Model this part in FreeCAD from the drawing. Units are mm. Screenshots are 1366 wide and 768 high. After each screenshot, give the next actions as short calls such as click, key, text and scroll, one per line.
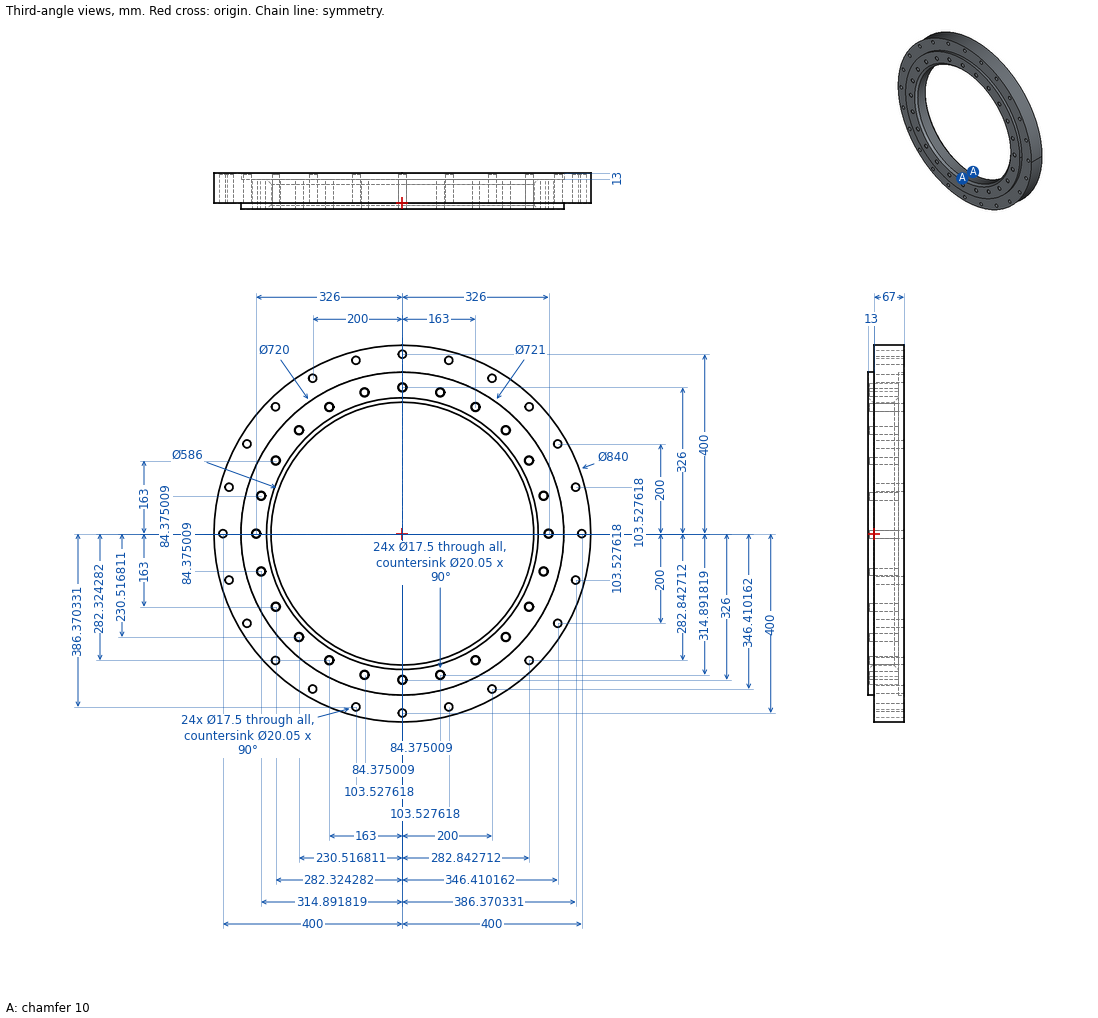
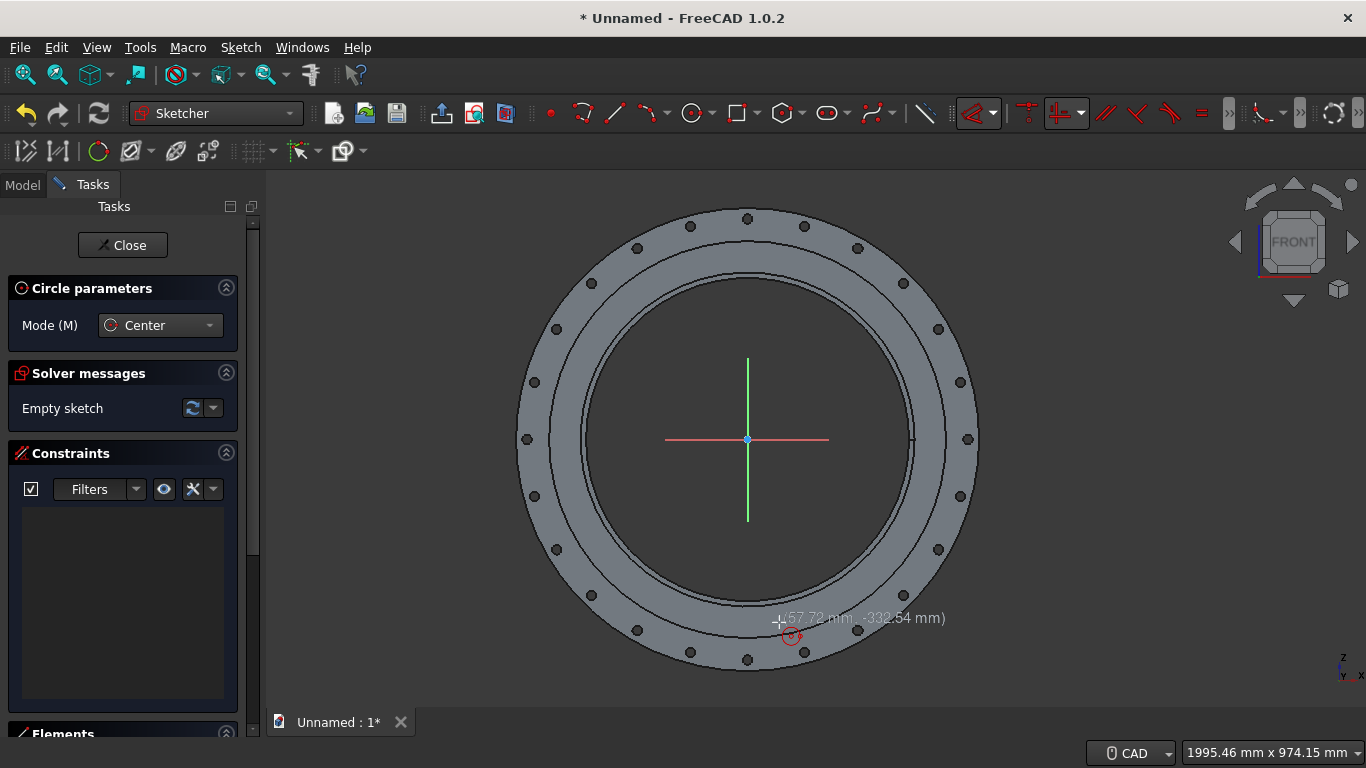
click(794, 613)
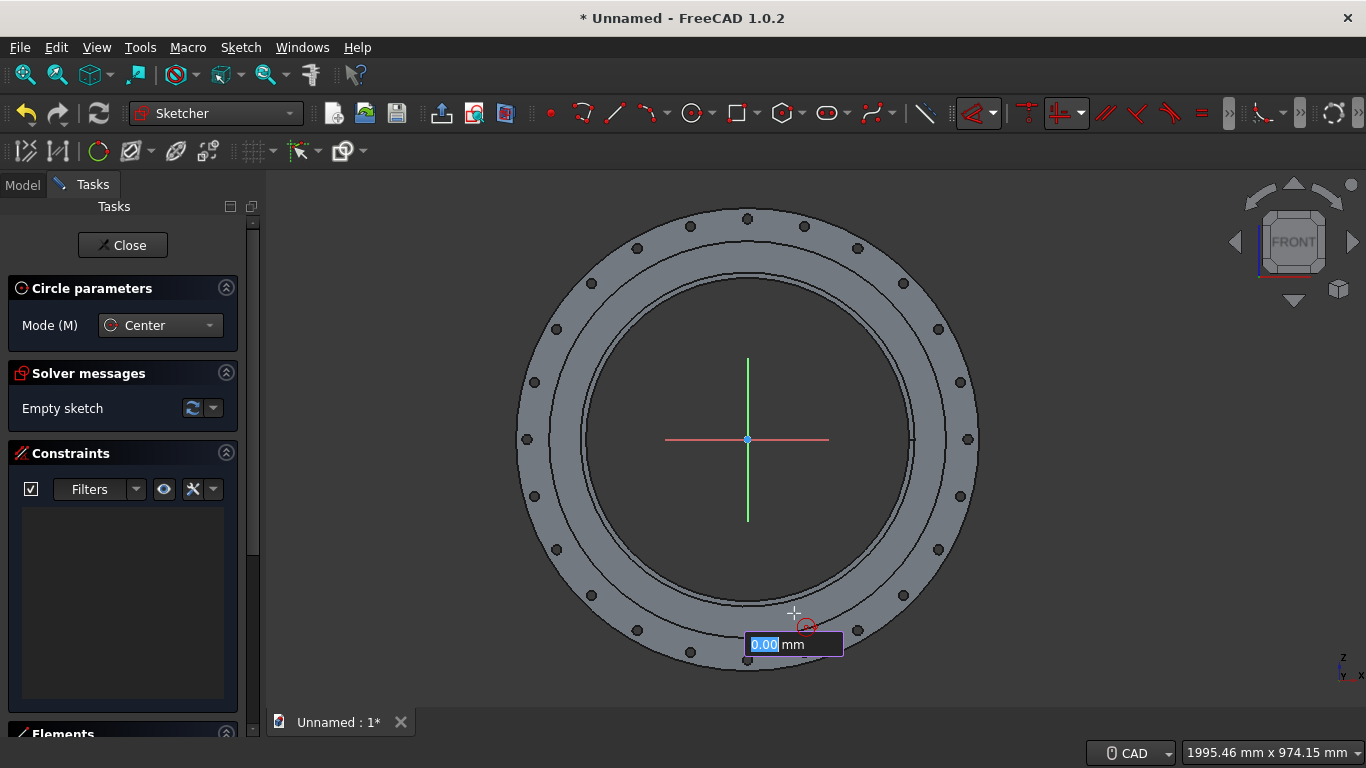
scroll(797, 610, up, 6)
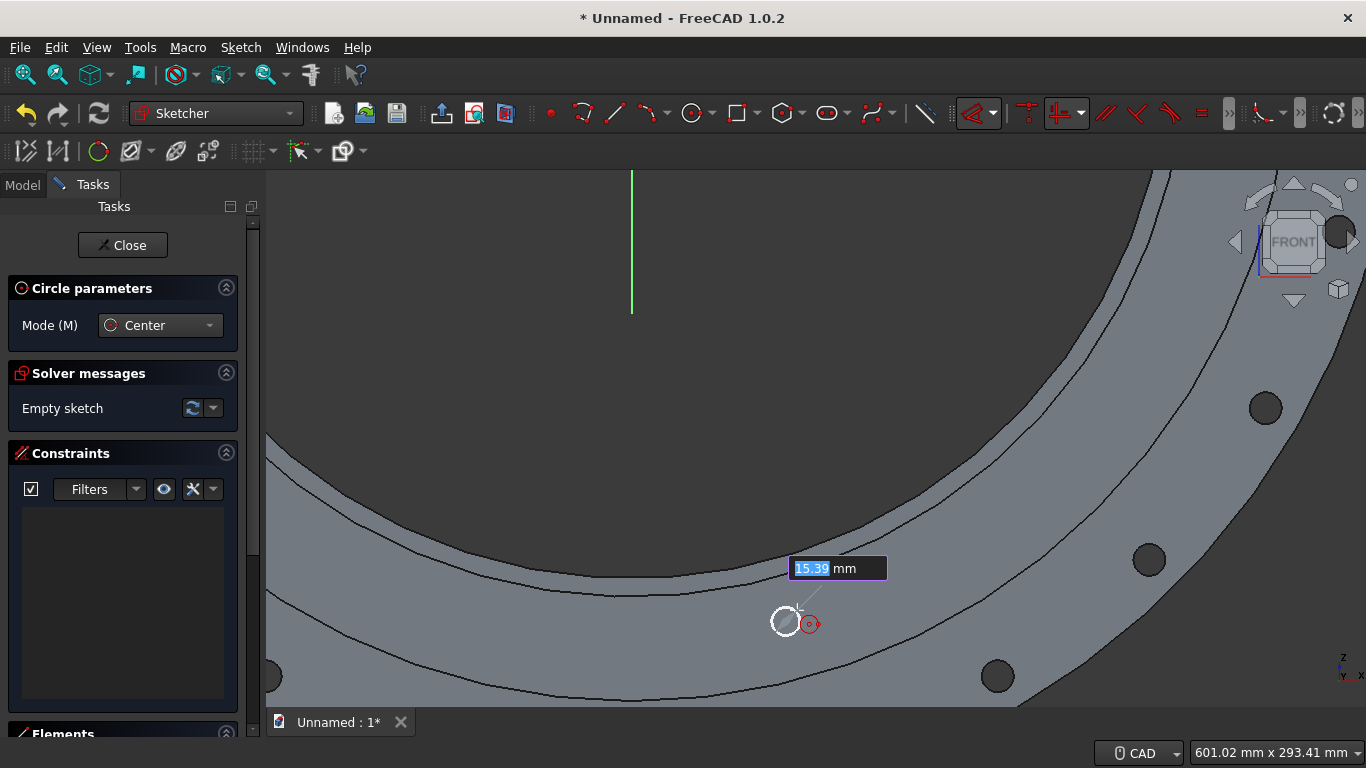
click(797, 607)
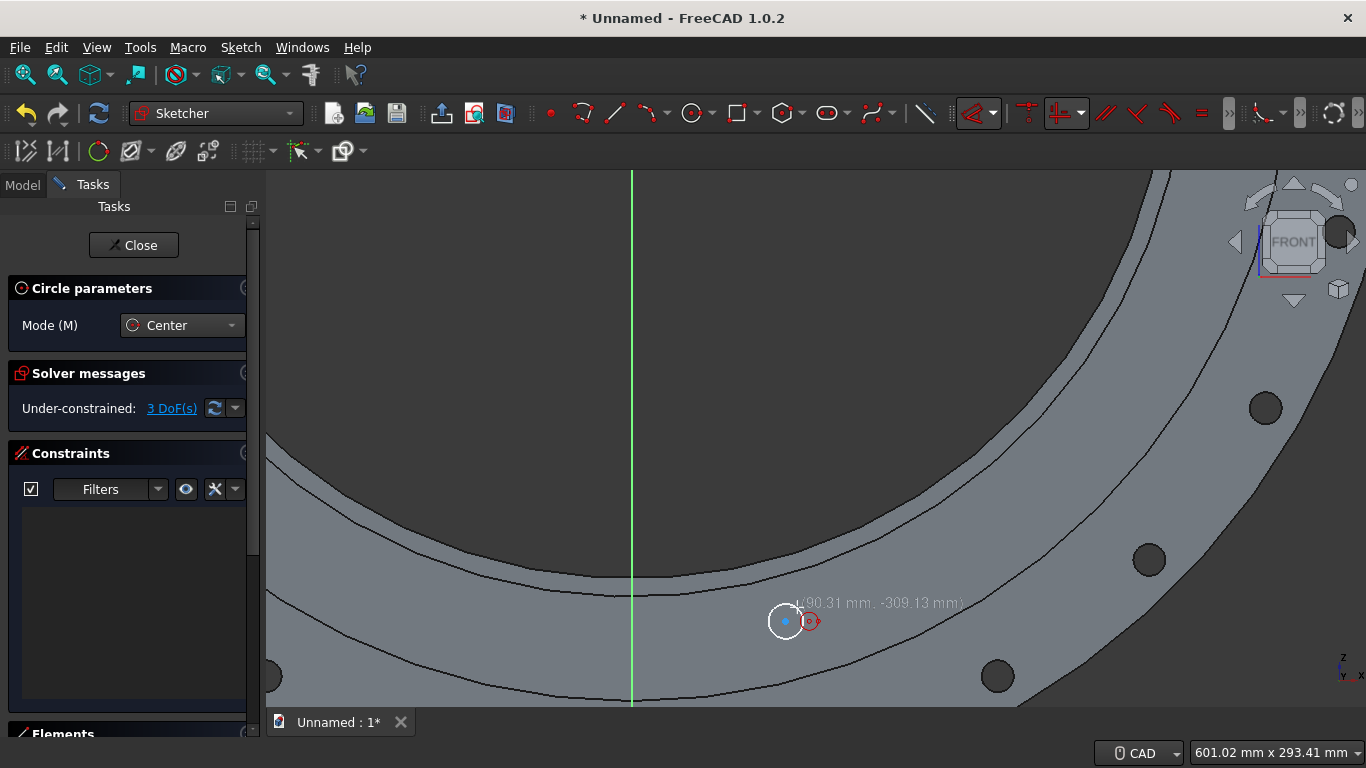
scroll(632, 639, up, 2)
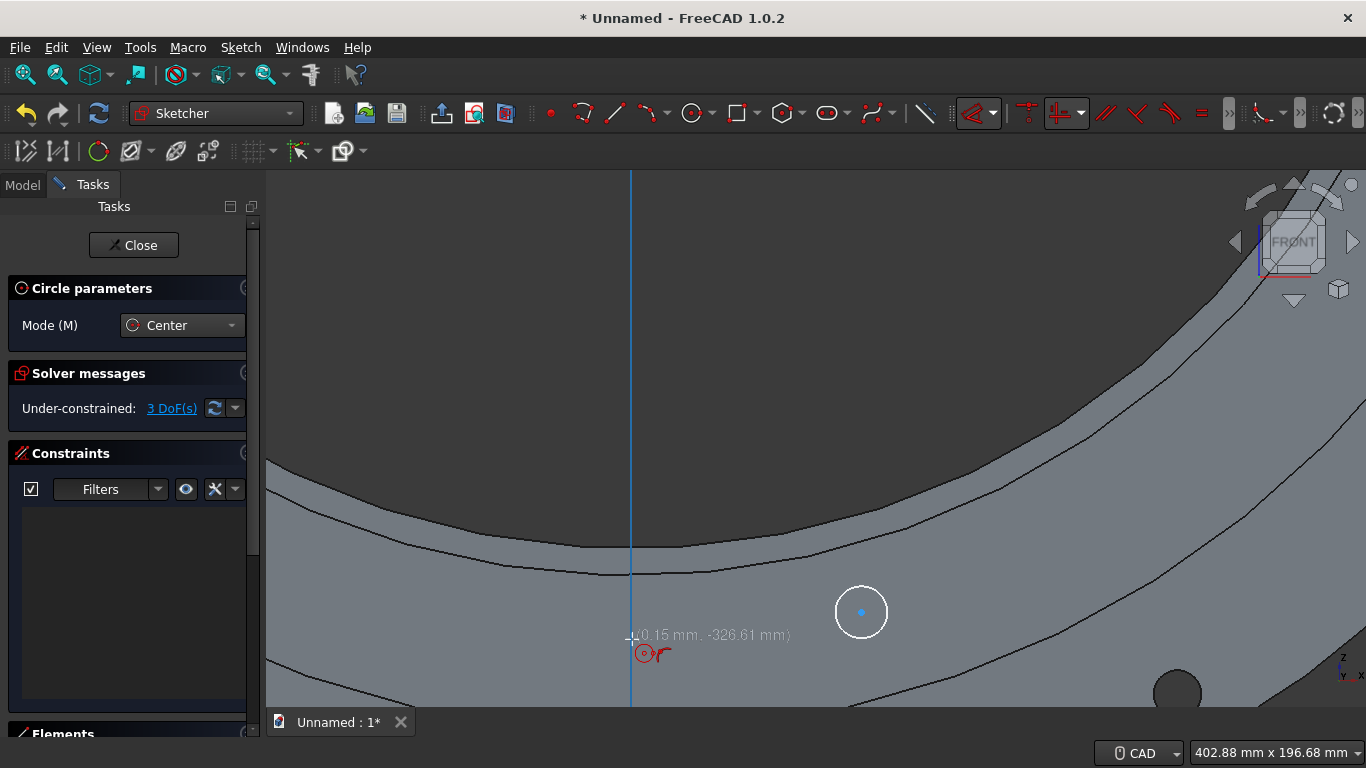
scroll(777, 613, down, 8)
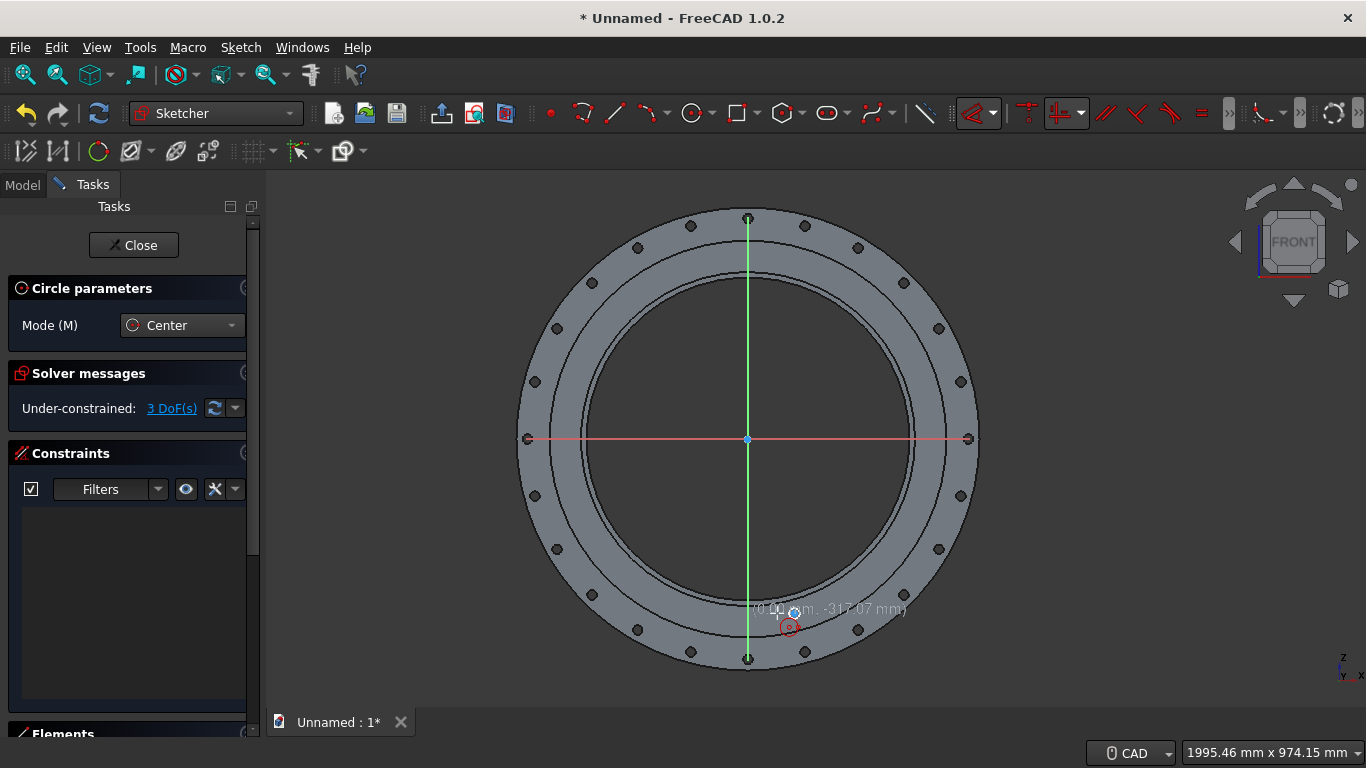
click(748, 619)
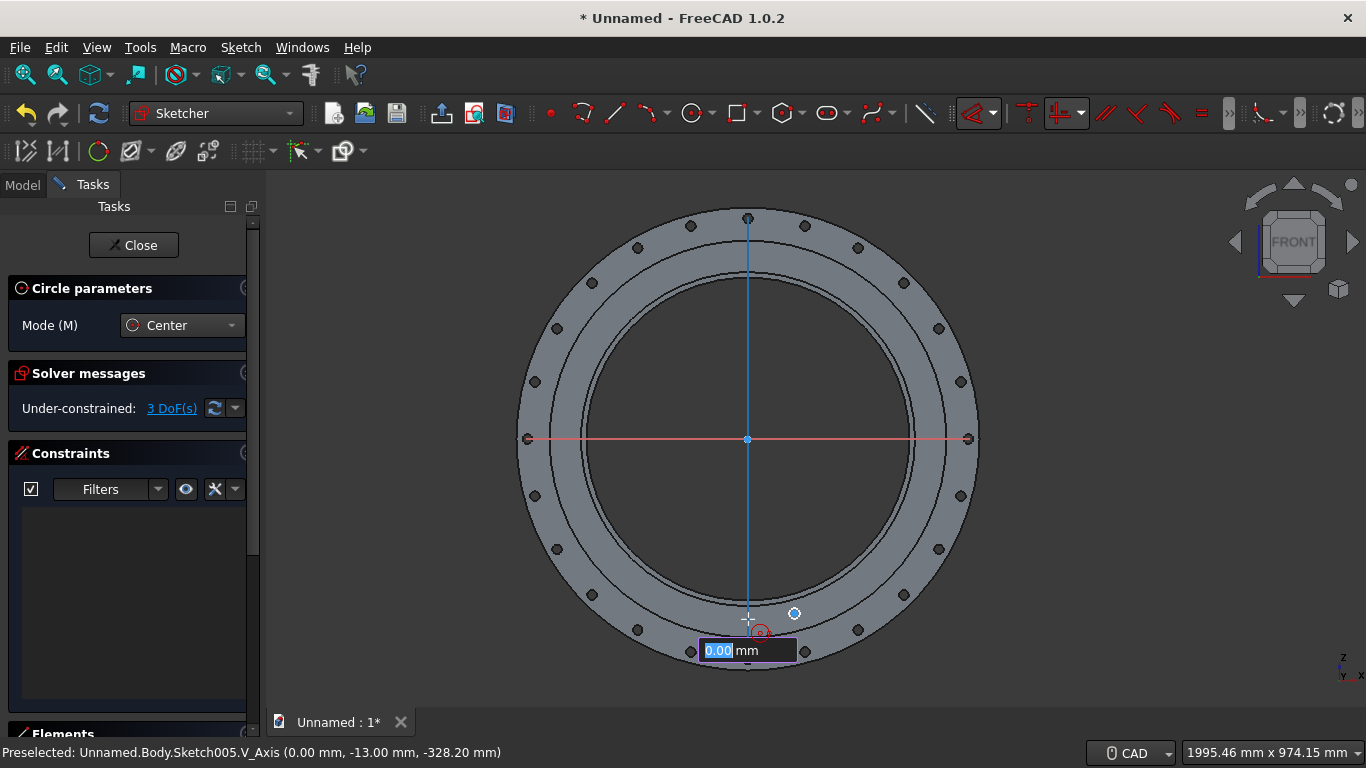
scroll(753, 617, up, 7)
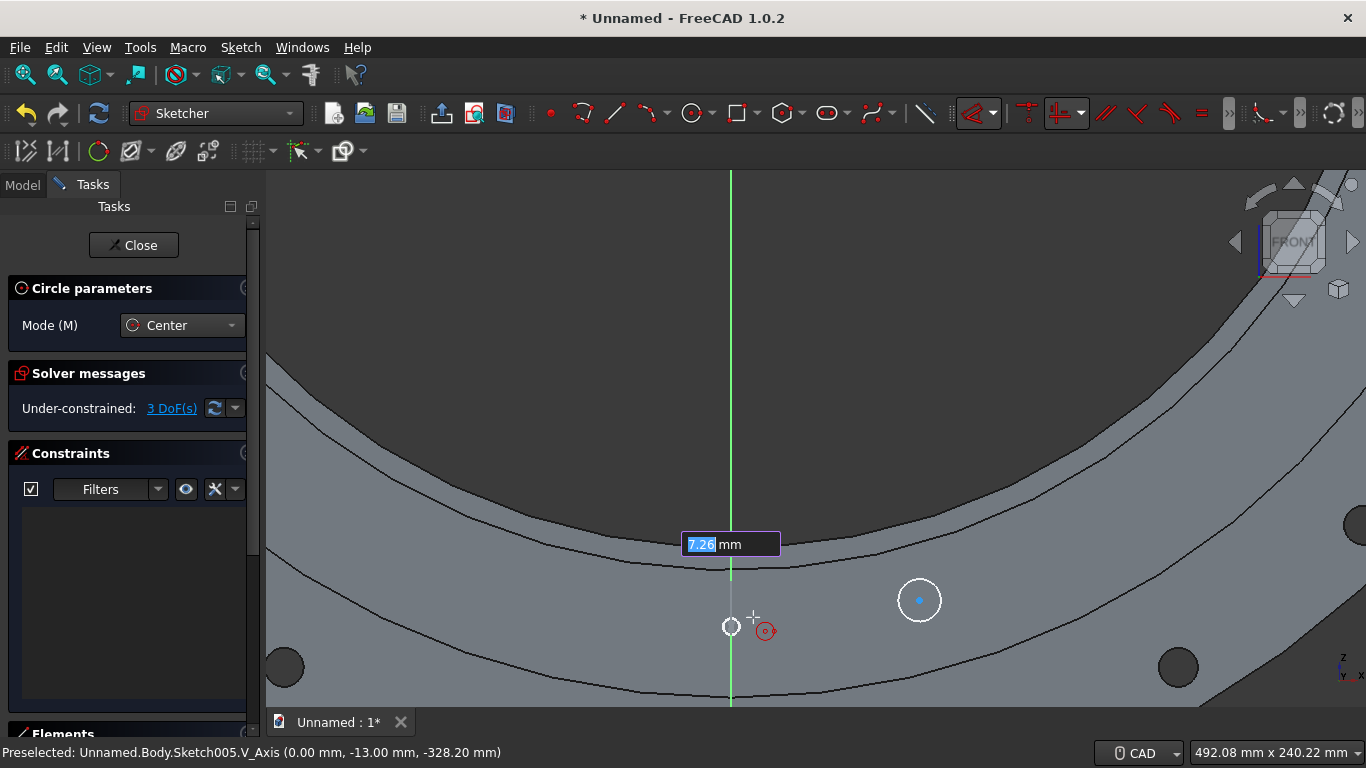
click(750, 615)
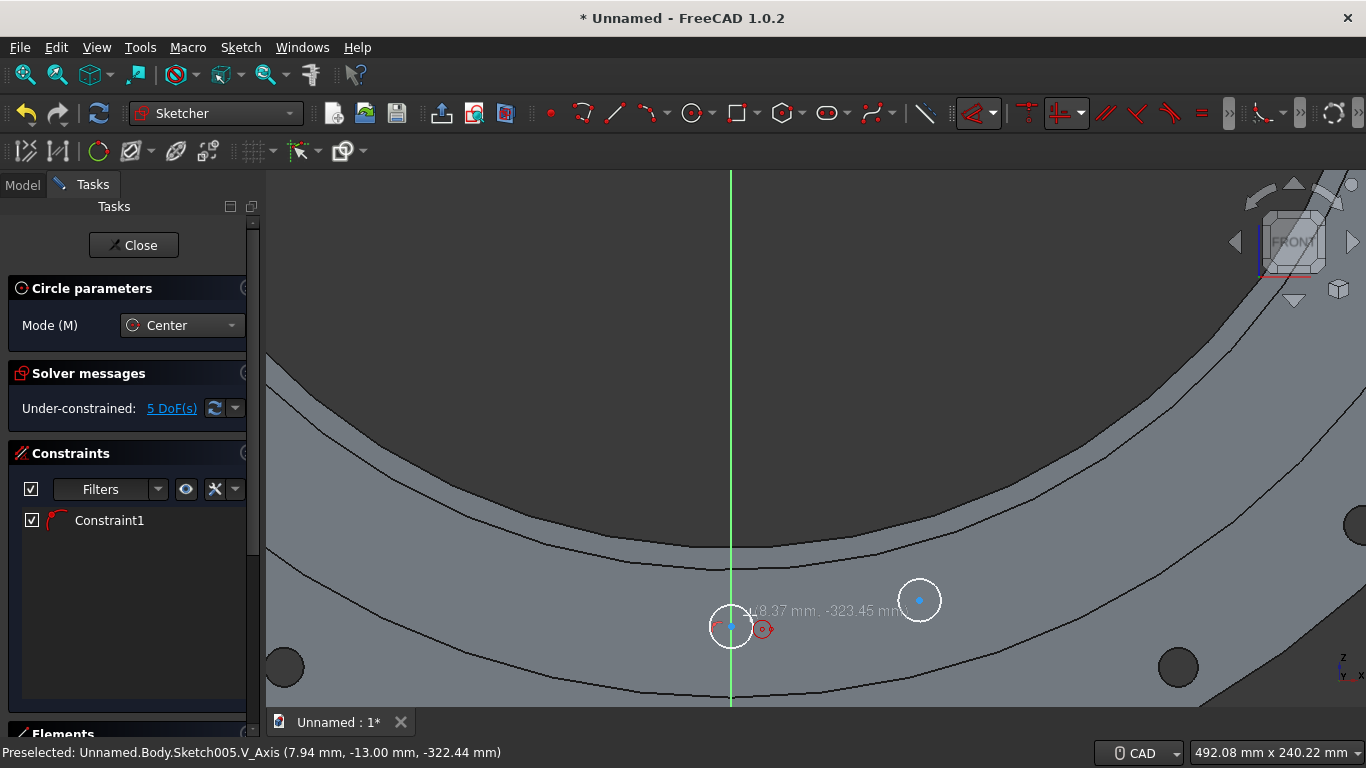
scroll(753, 617, down, 7)